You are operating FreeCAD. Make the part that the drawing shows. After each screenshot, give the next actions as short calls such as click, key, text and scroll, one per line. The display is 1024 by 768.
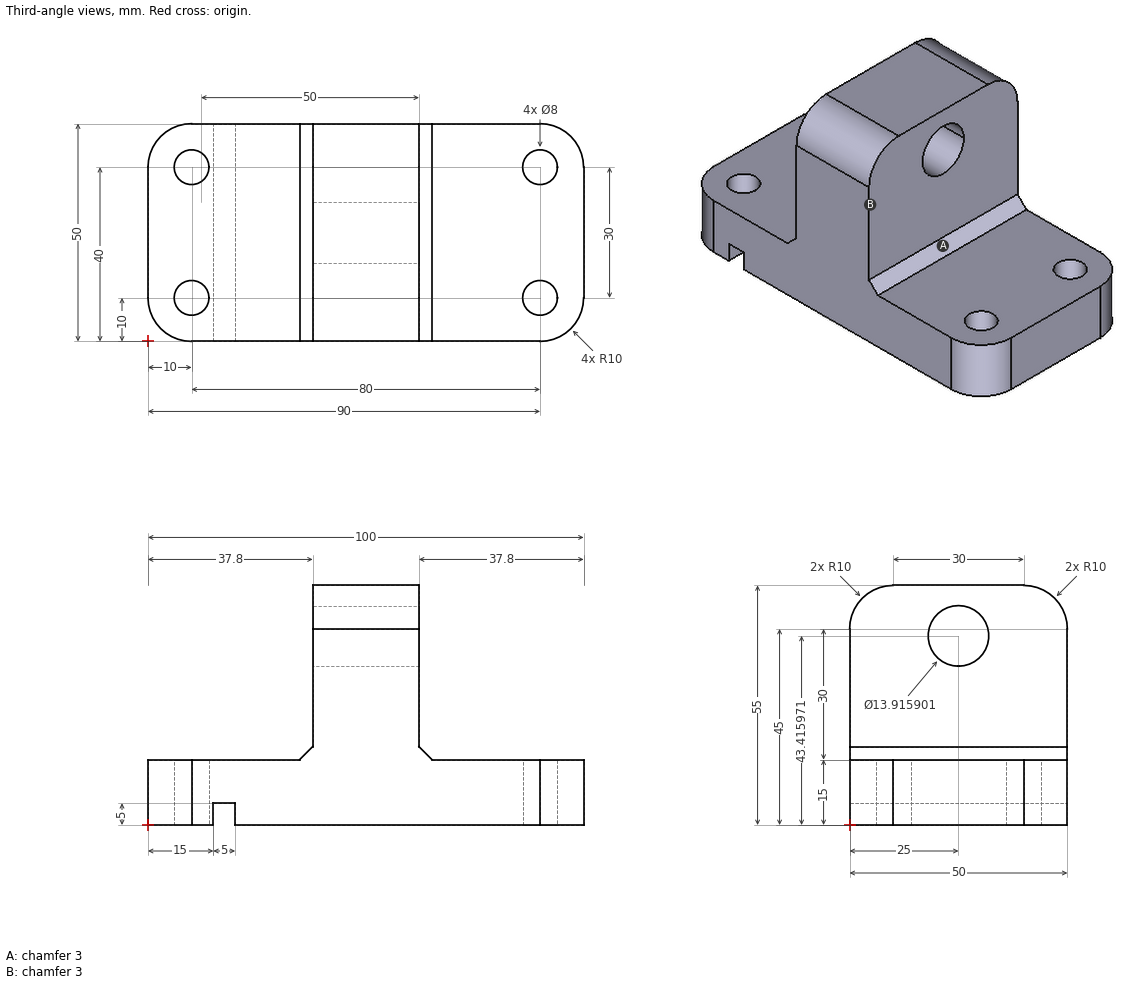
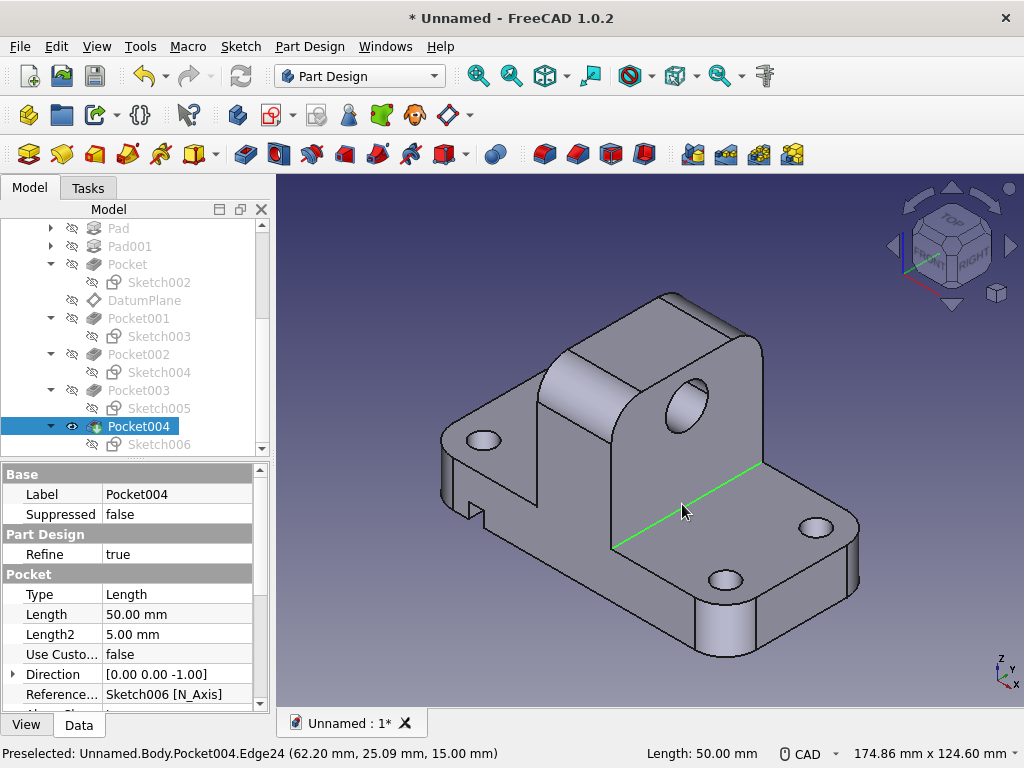
click(578, 154)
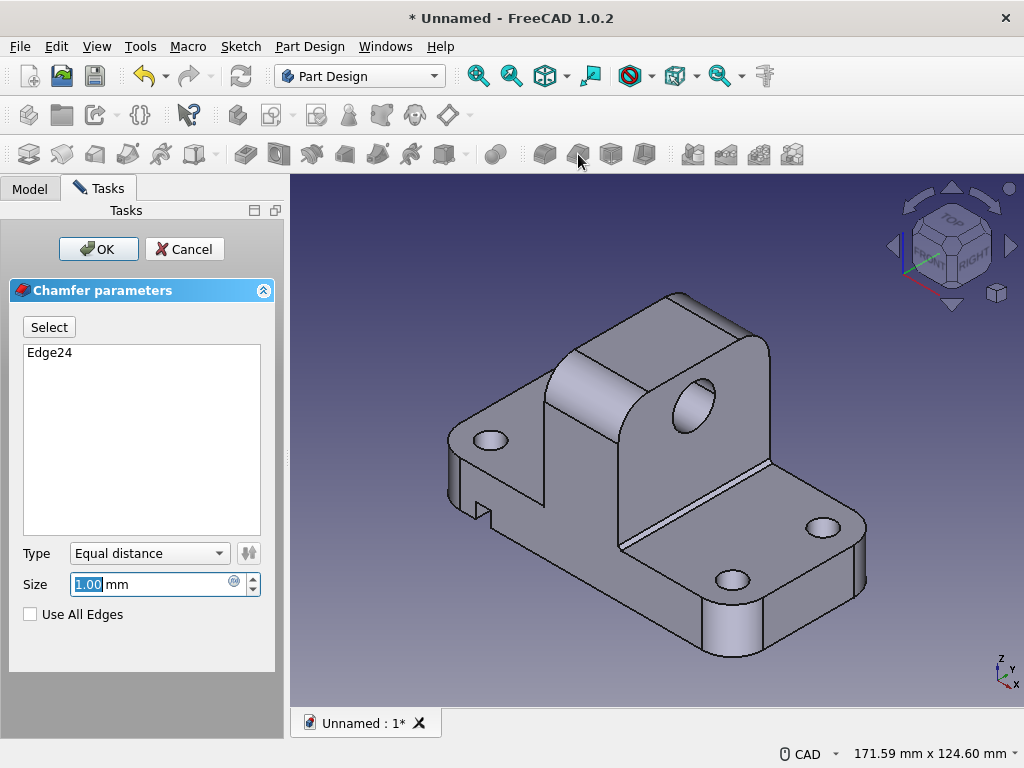
text(3)
key(Tab)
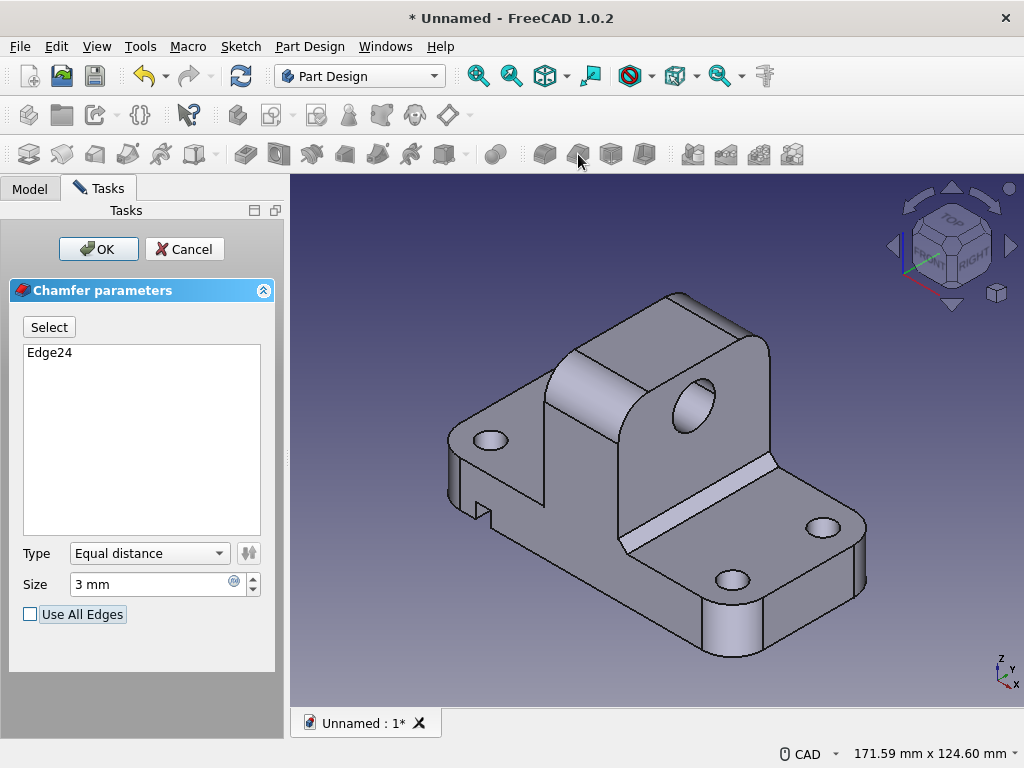
click(99, 249)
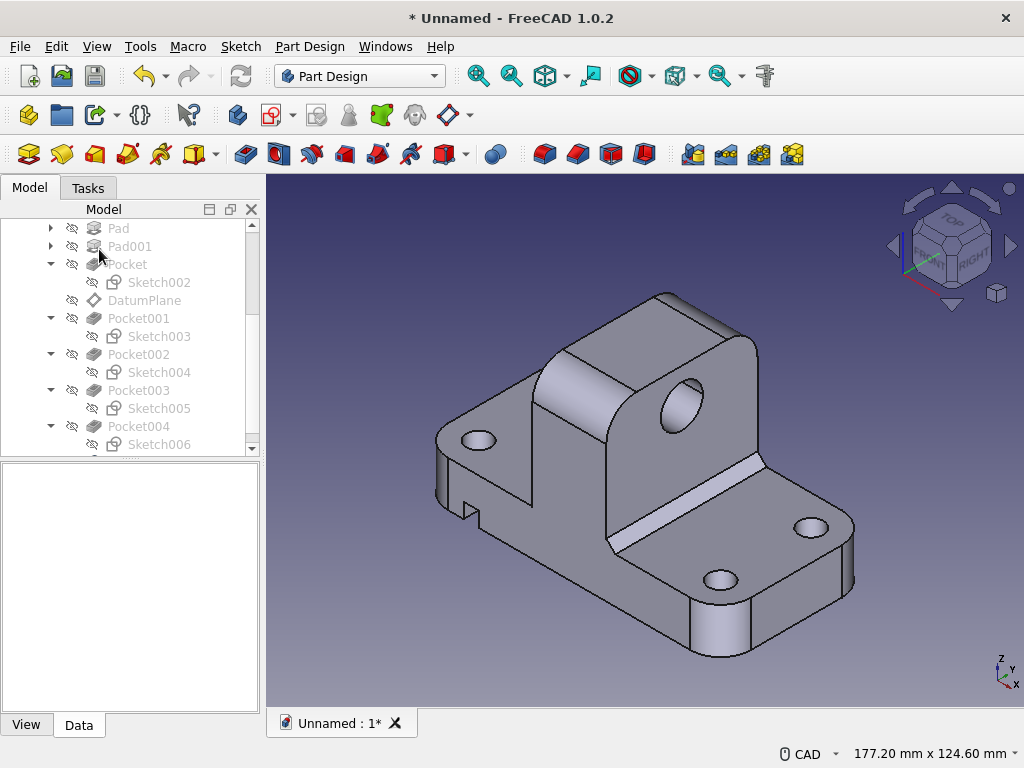
key(2)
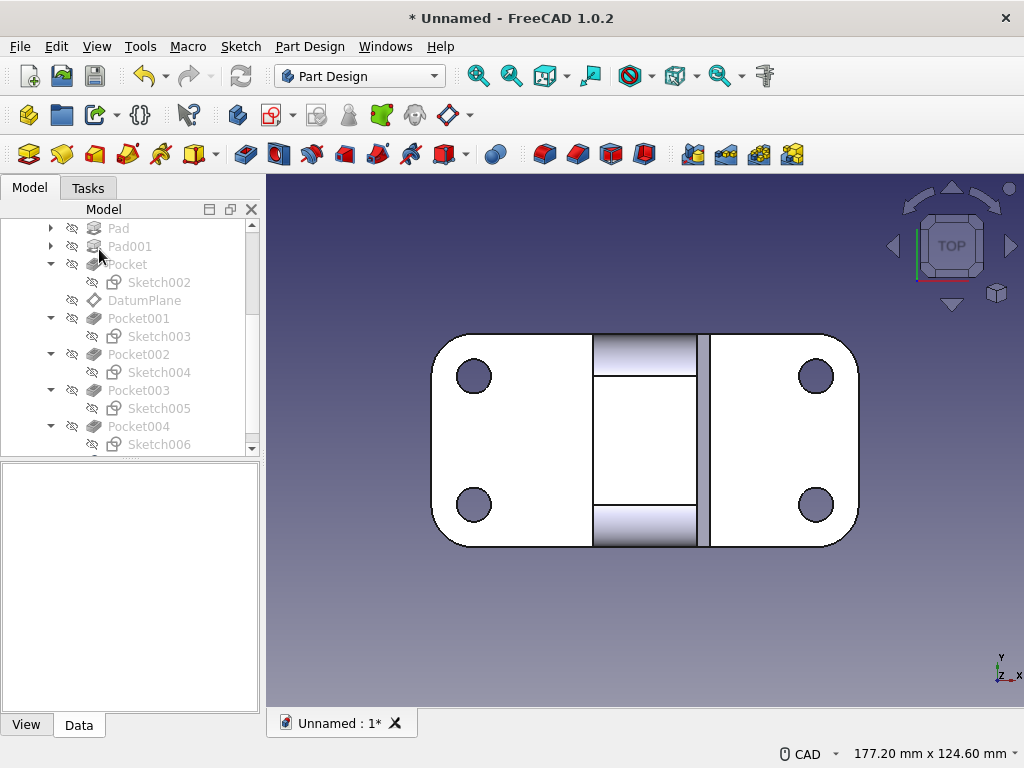
key(0)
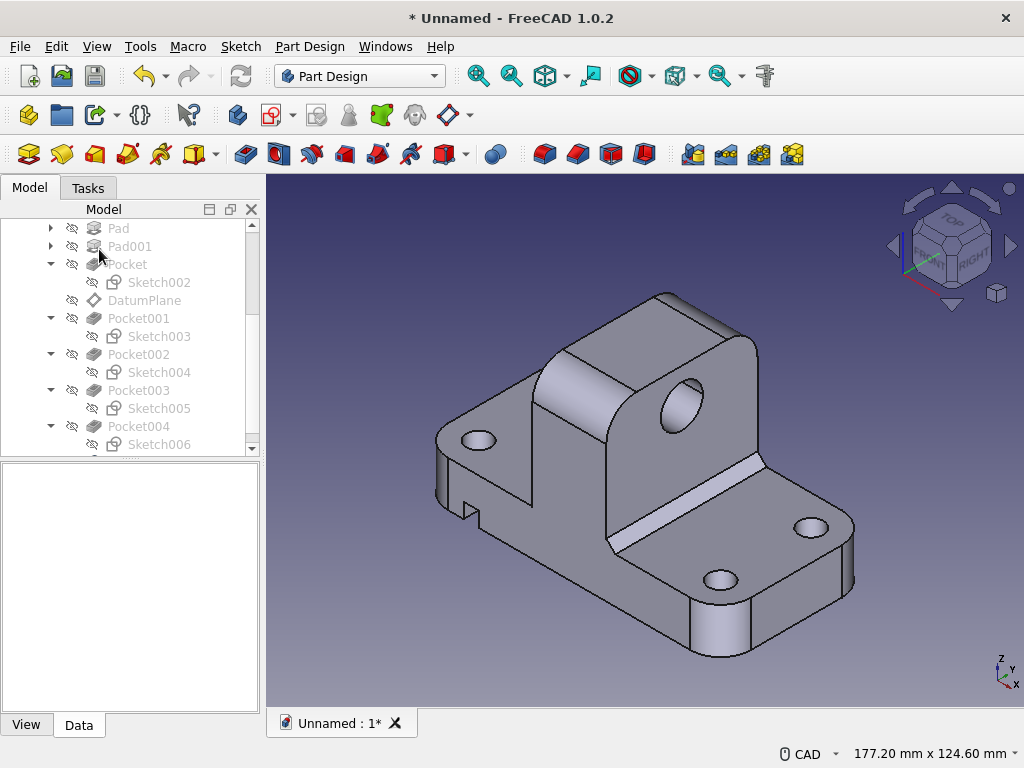
key(1)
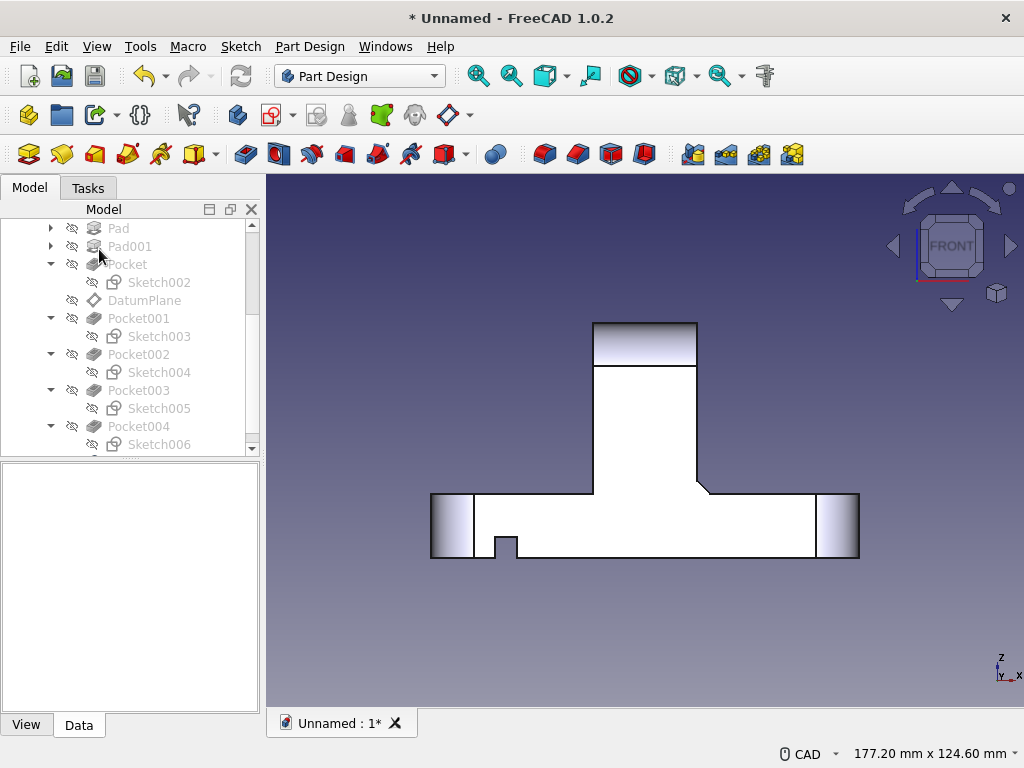
key(3)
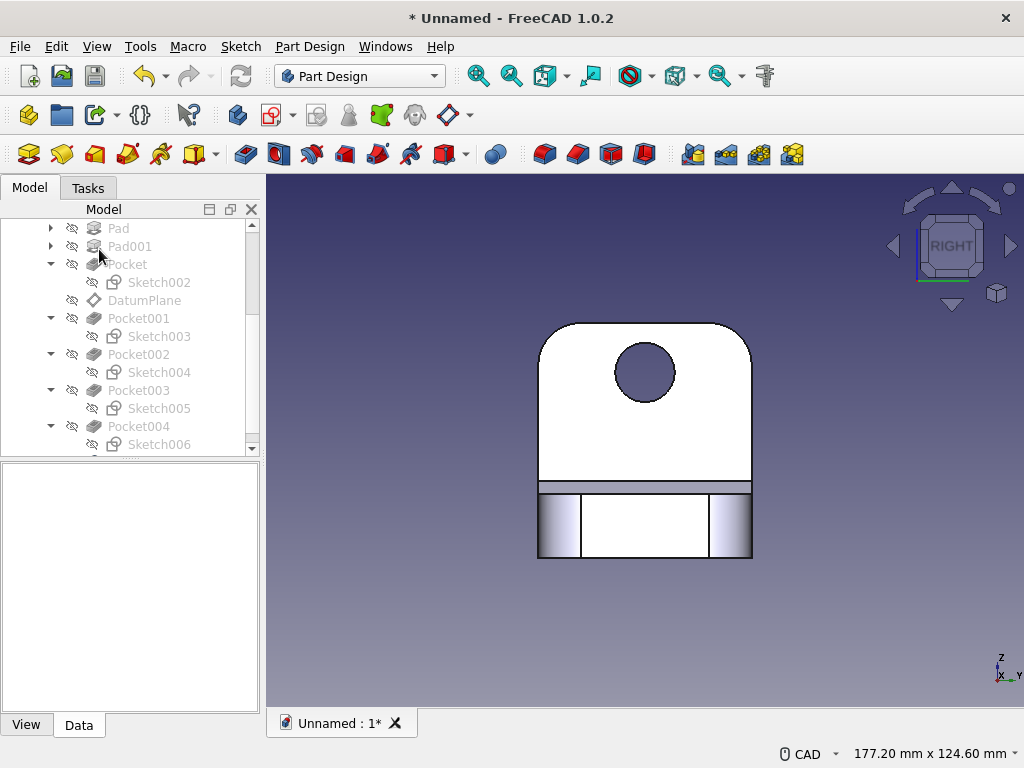
click(479, 76)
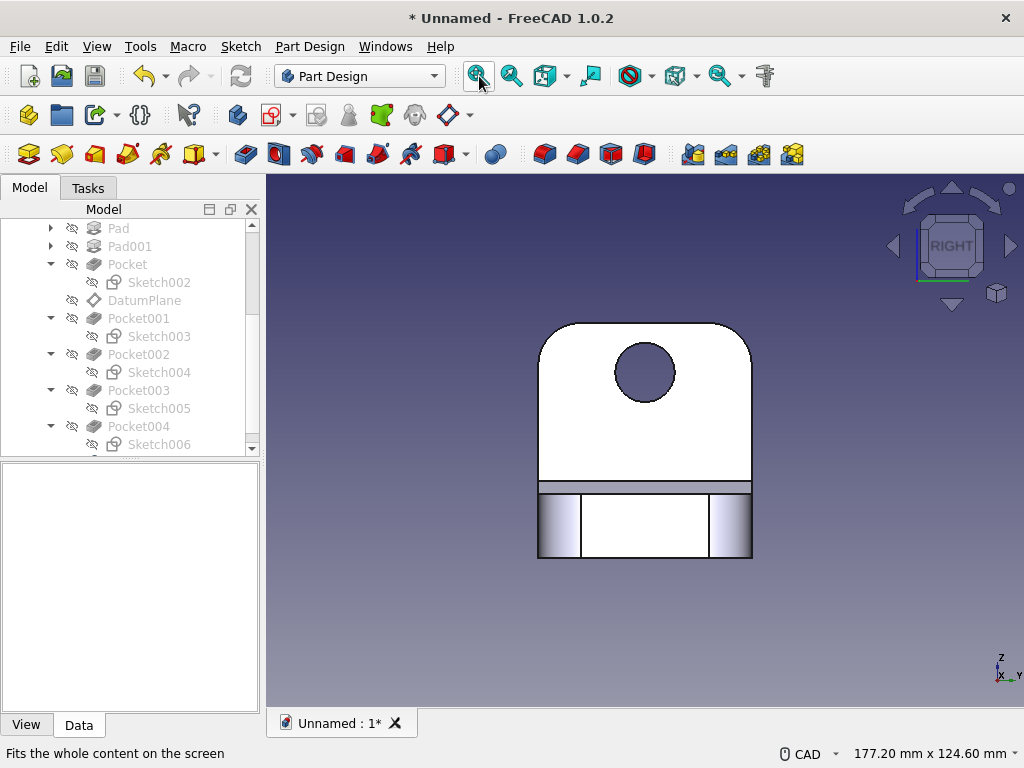
key(5)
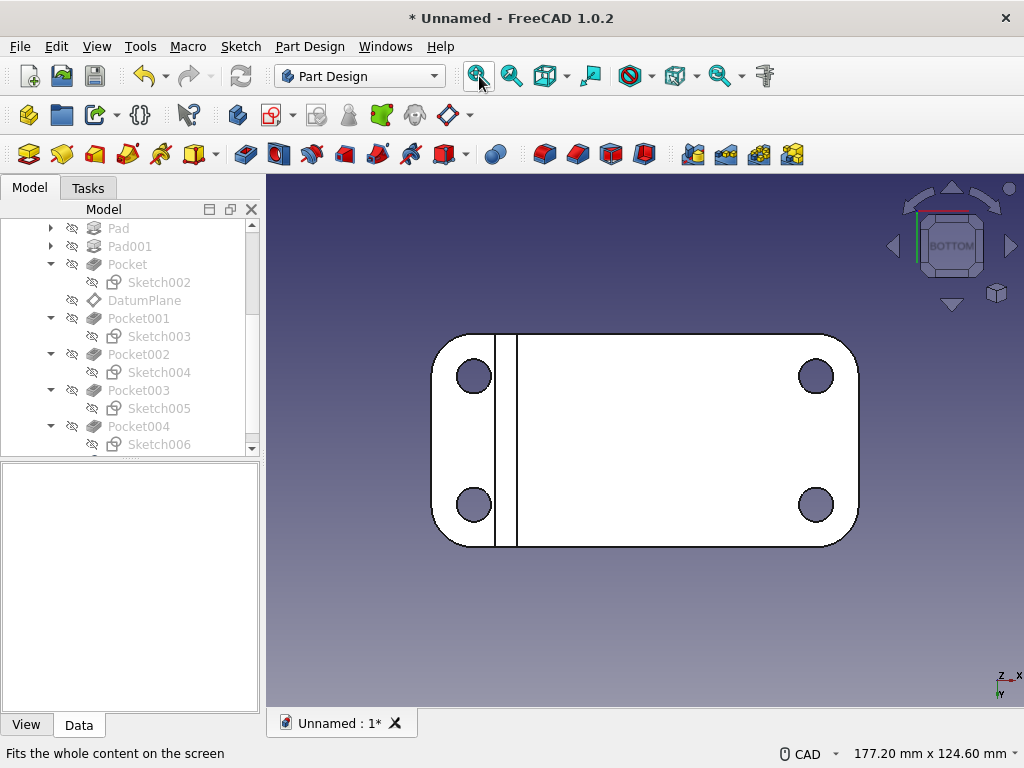
key(4)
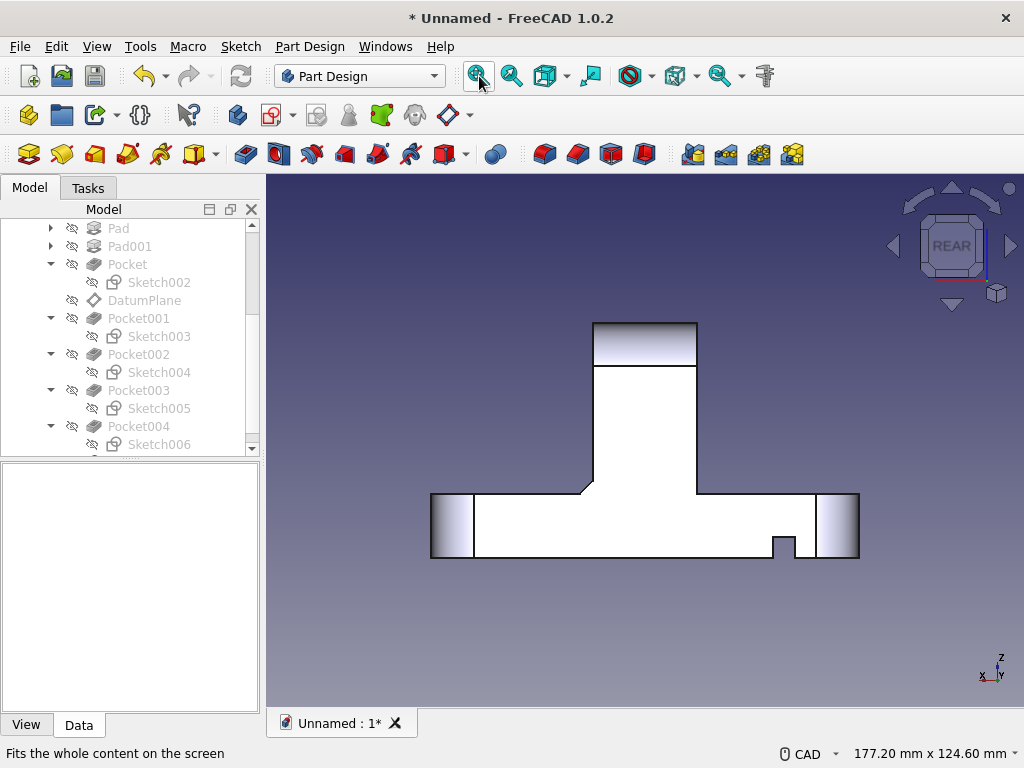
key(6)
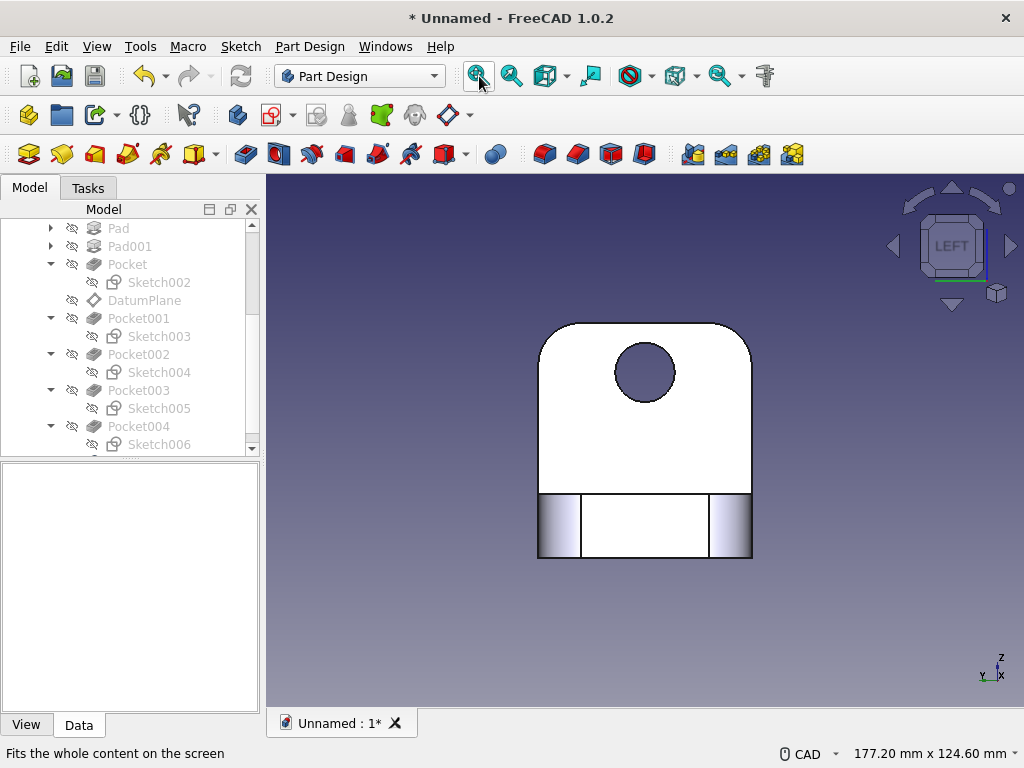
click(479, 76)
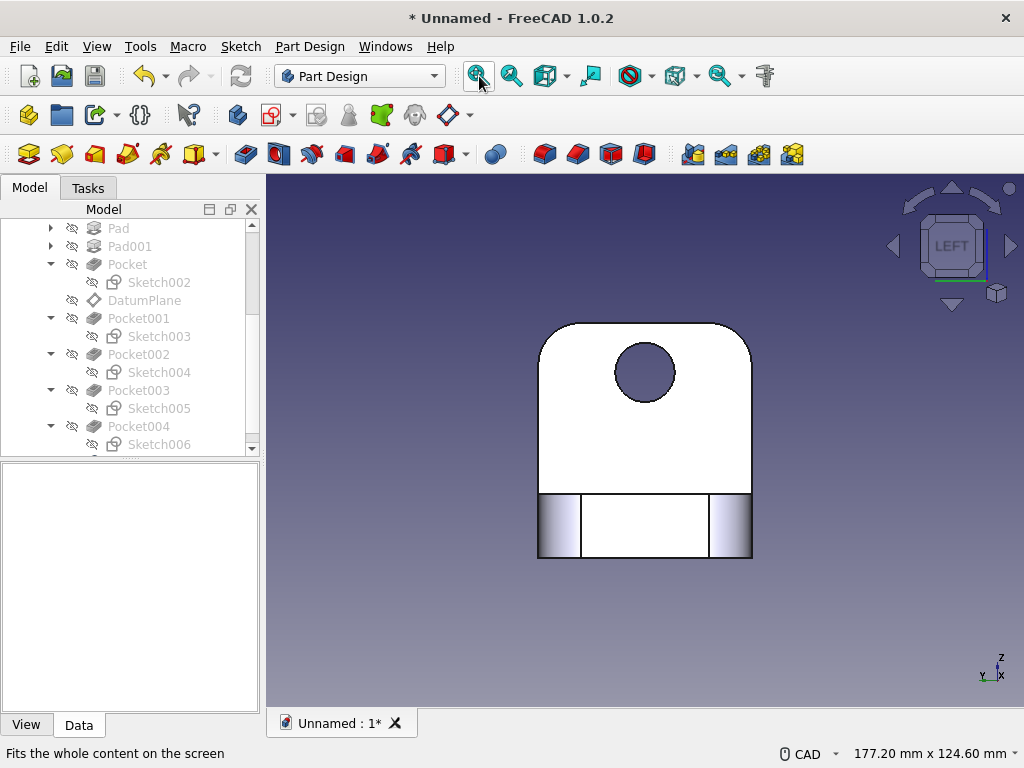
key(v)
key(3)